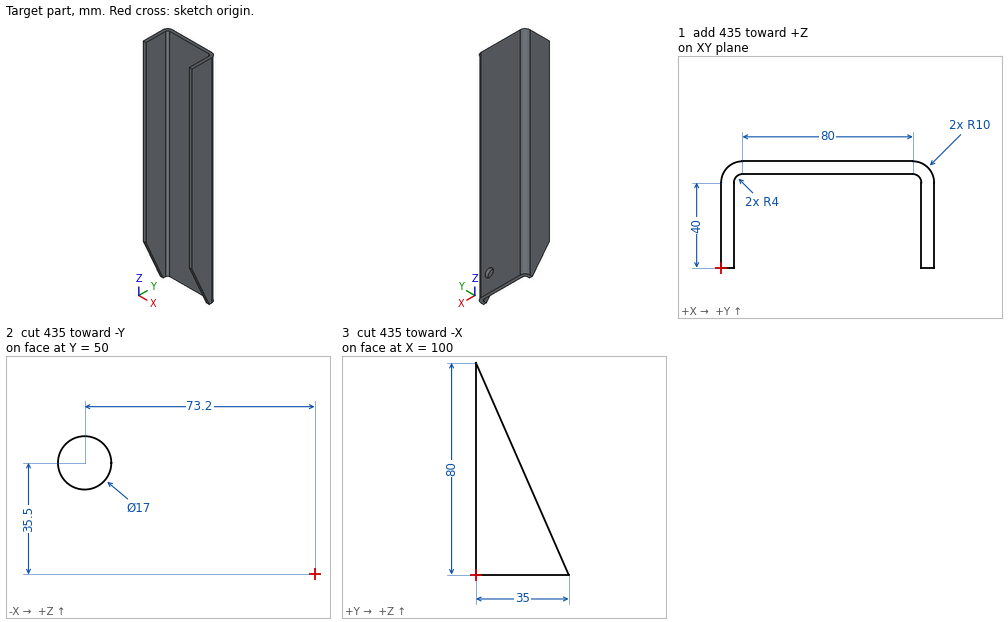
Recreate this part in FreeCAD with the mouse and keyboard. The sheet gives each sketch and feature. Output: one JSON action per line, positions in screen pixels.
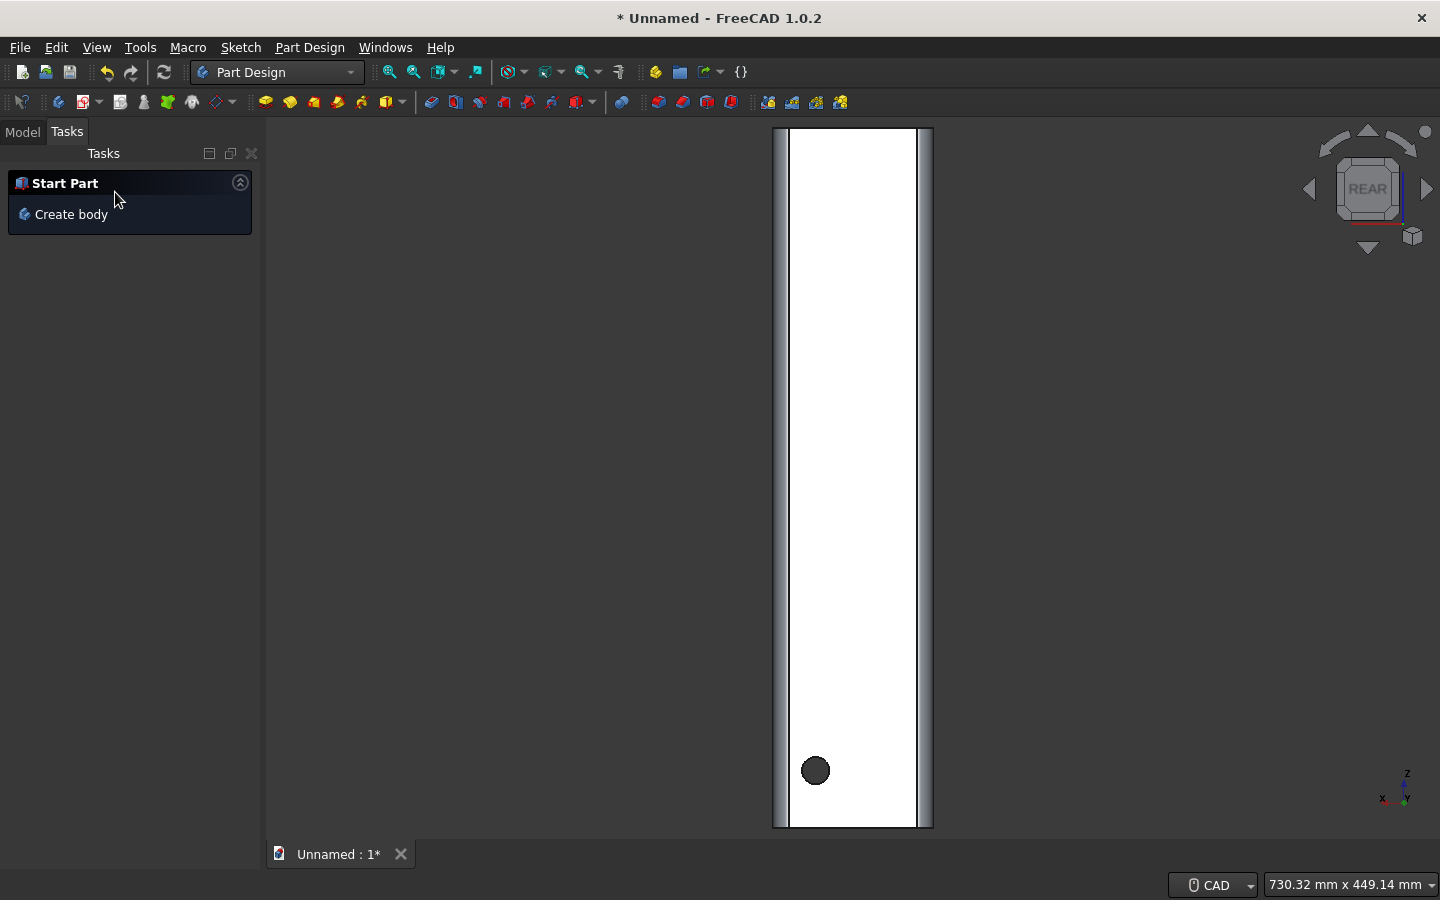
{"action": "key", "text": "0"}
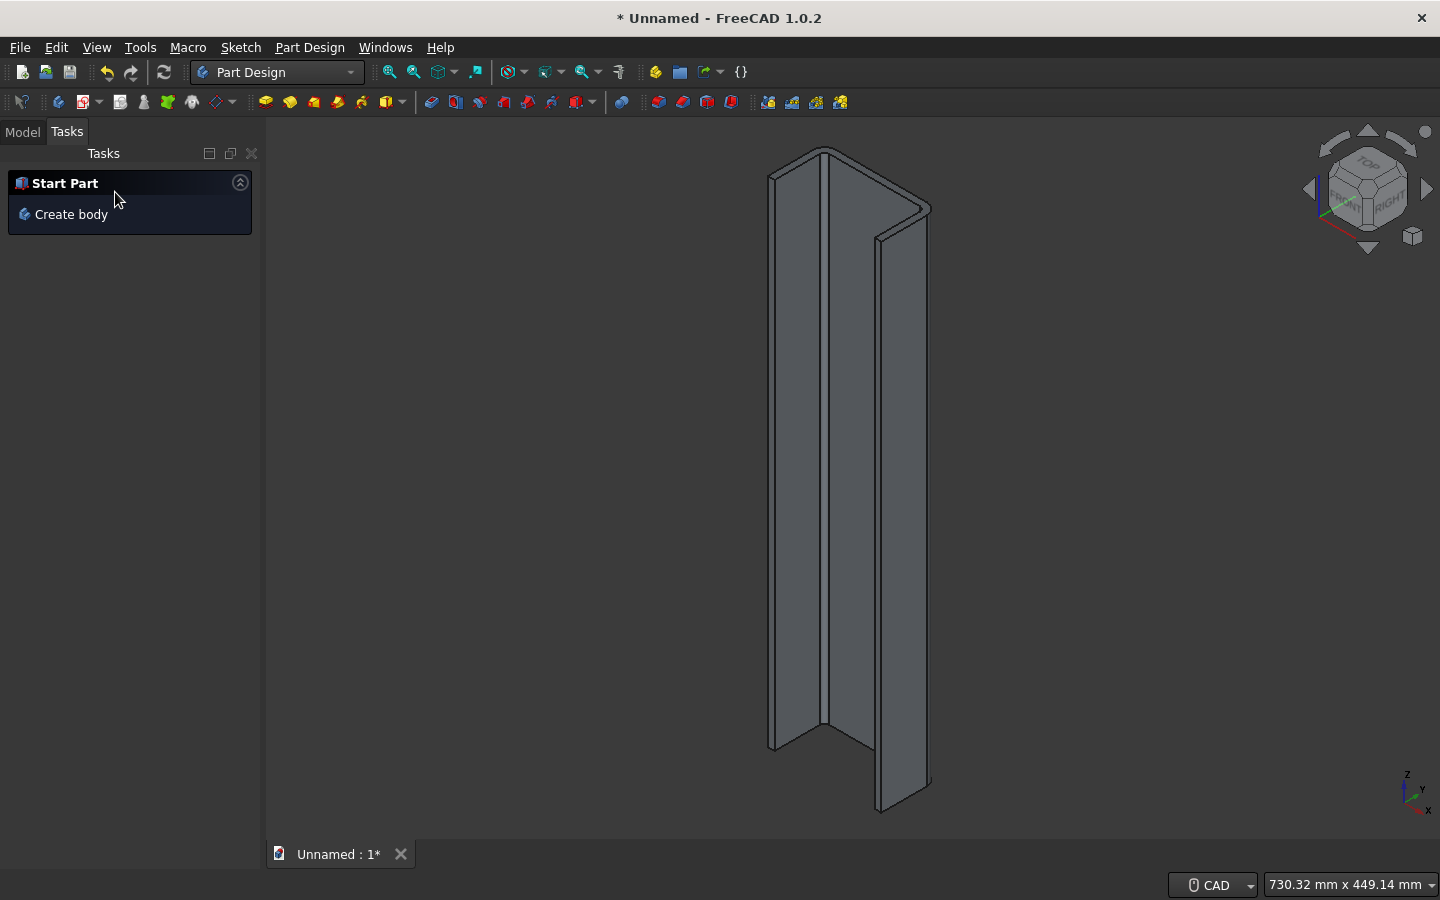
{"action": "left_click", "coordinate": [904, 268]}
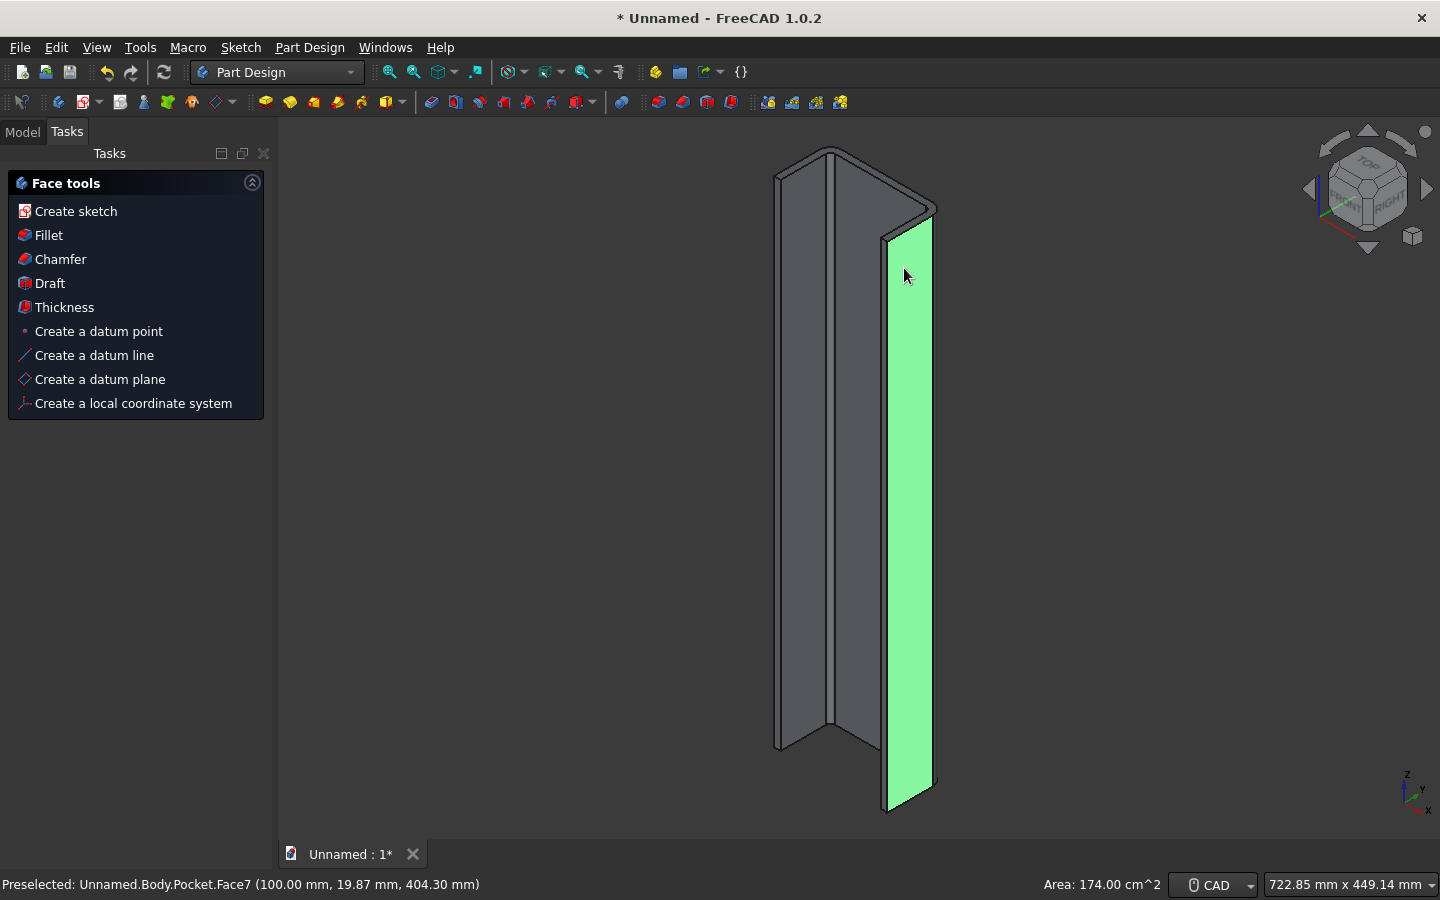
{"action": "left_click", "coordinate": [84, 102]}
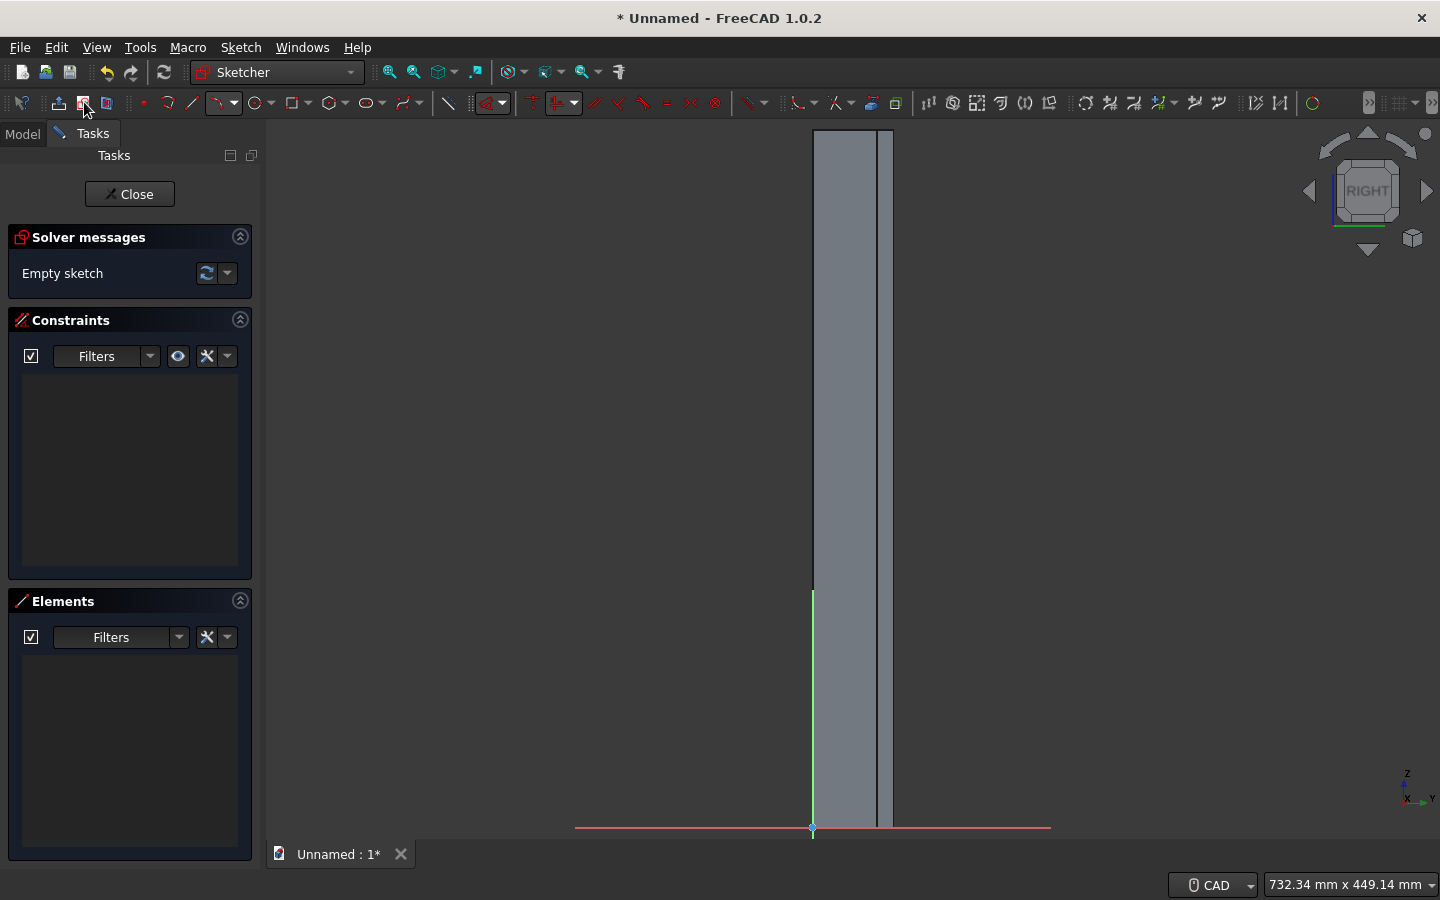
{"action": "scroll", "coordinate": [784, 479], "scroll_direction": "down", "scroll_amount": 5}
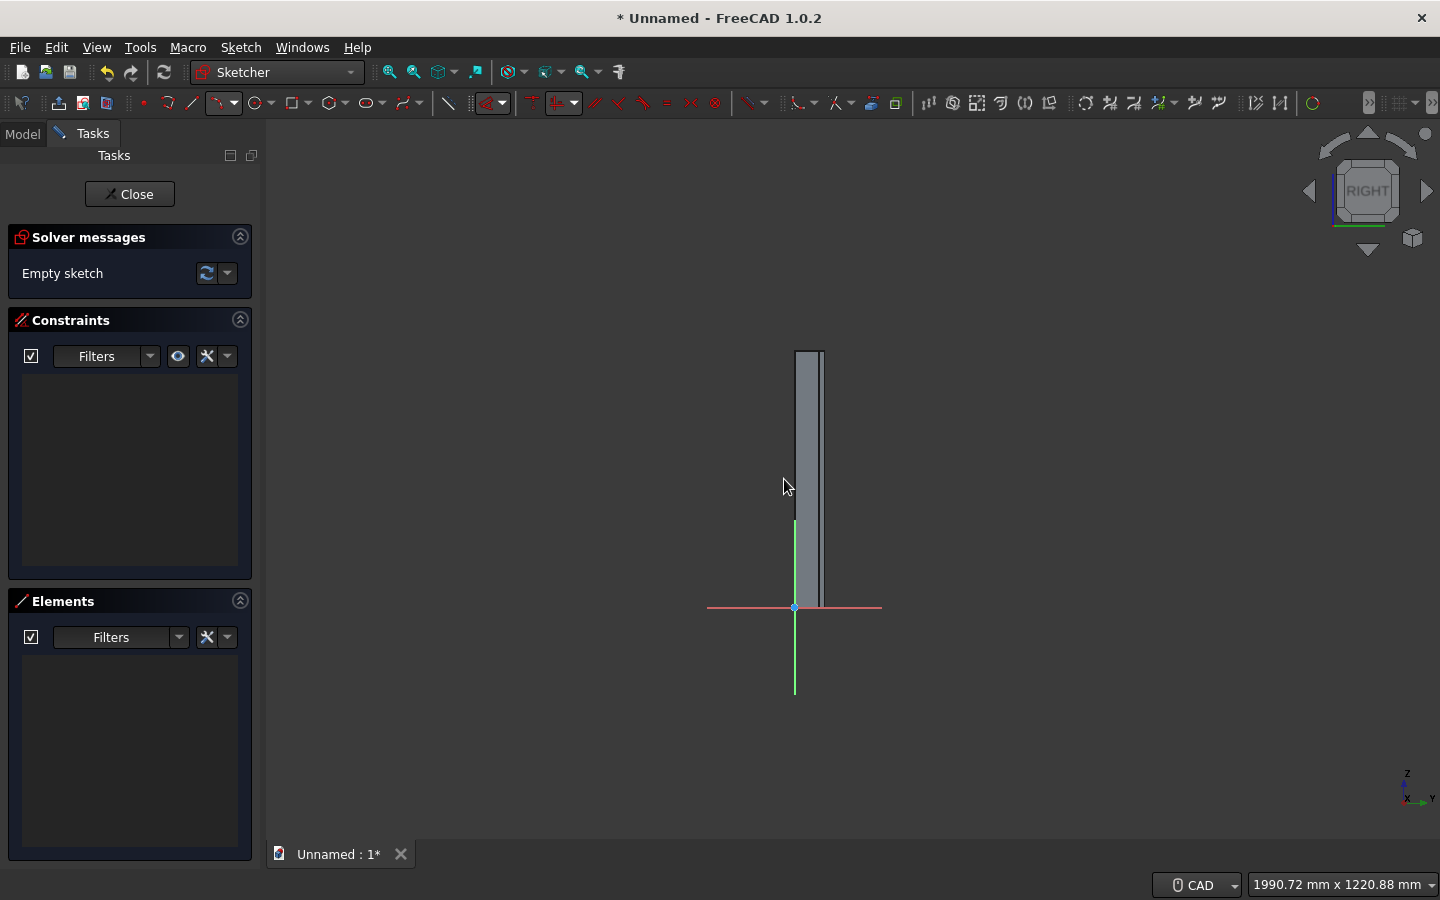
{"action": "scroll", "coordinate": [808, 597], "scroll_direction": "up", "scroll_amount": 11}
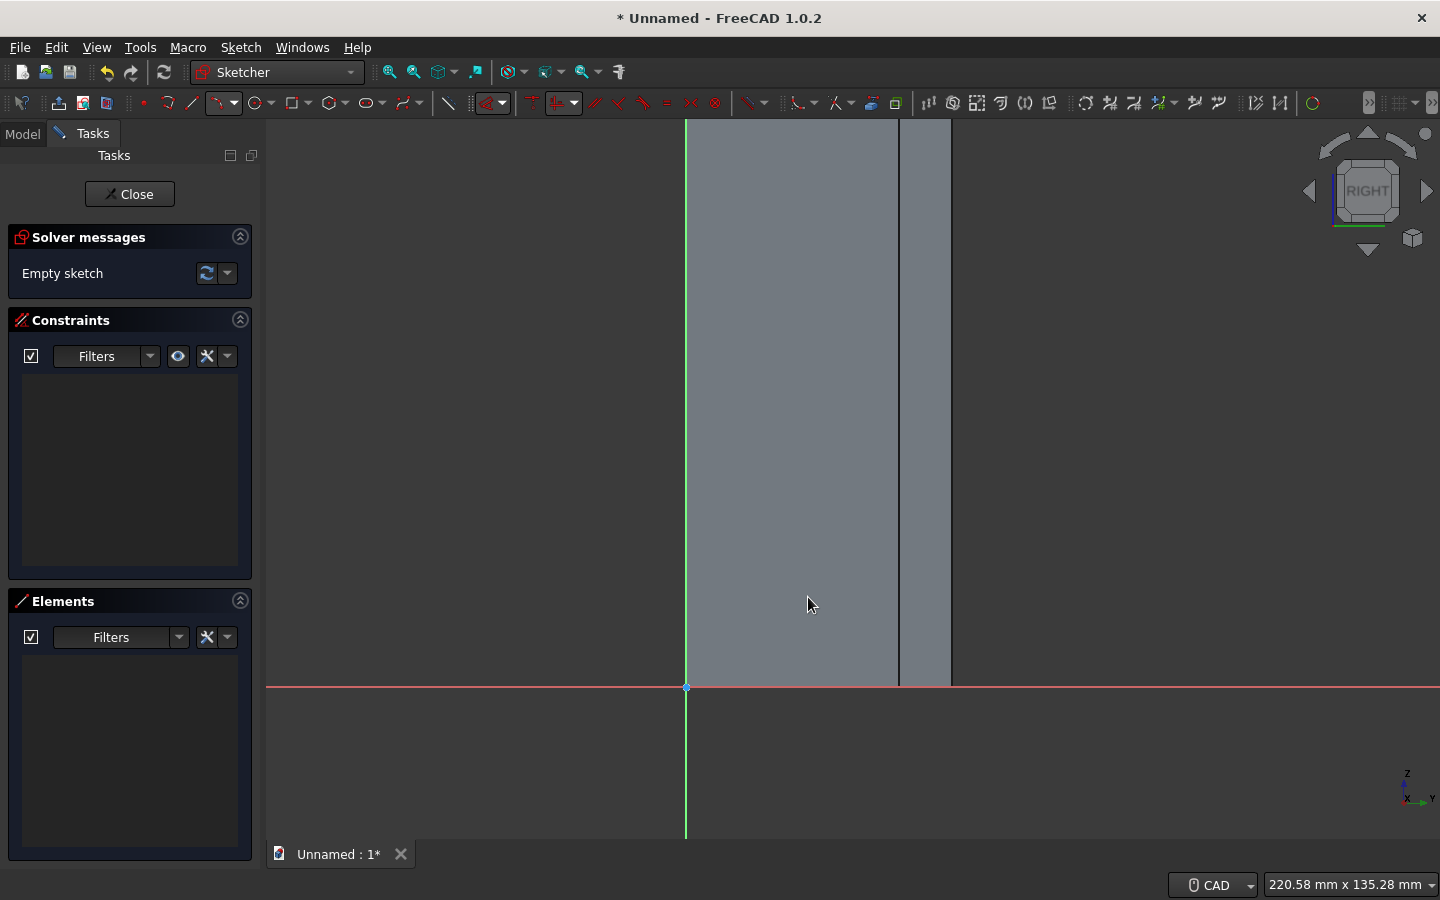
{"action": "left_click", "coordinate": [168, 104]}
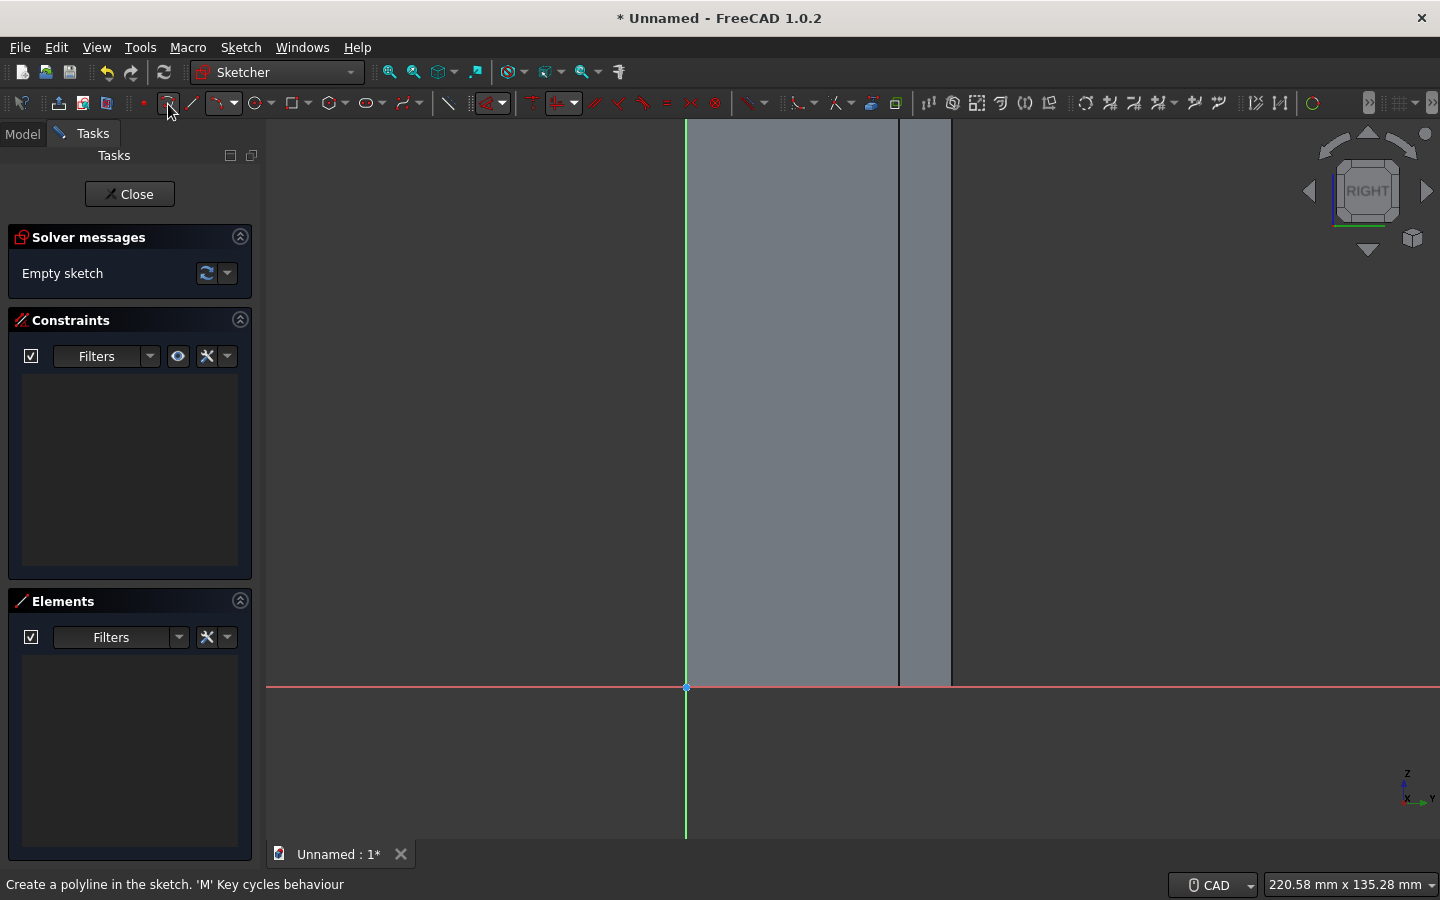
{"action": "left_click", "coordinate": [686, 687]}
{"action": "left_click", "coordinate": [873, 678]}
{"action": "left_click", "coordinate": [695, 261]}
{"action": "left_click", "coordinate": [686, 687]}
{"action": "key", "text": "Escape"}
{"action": "key", "text": "Escape"}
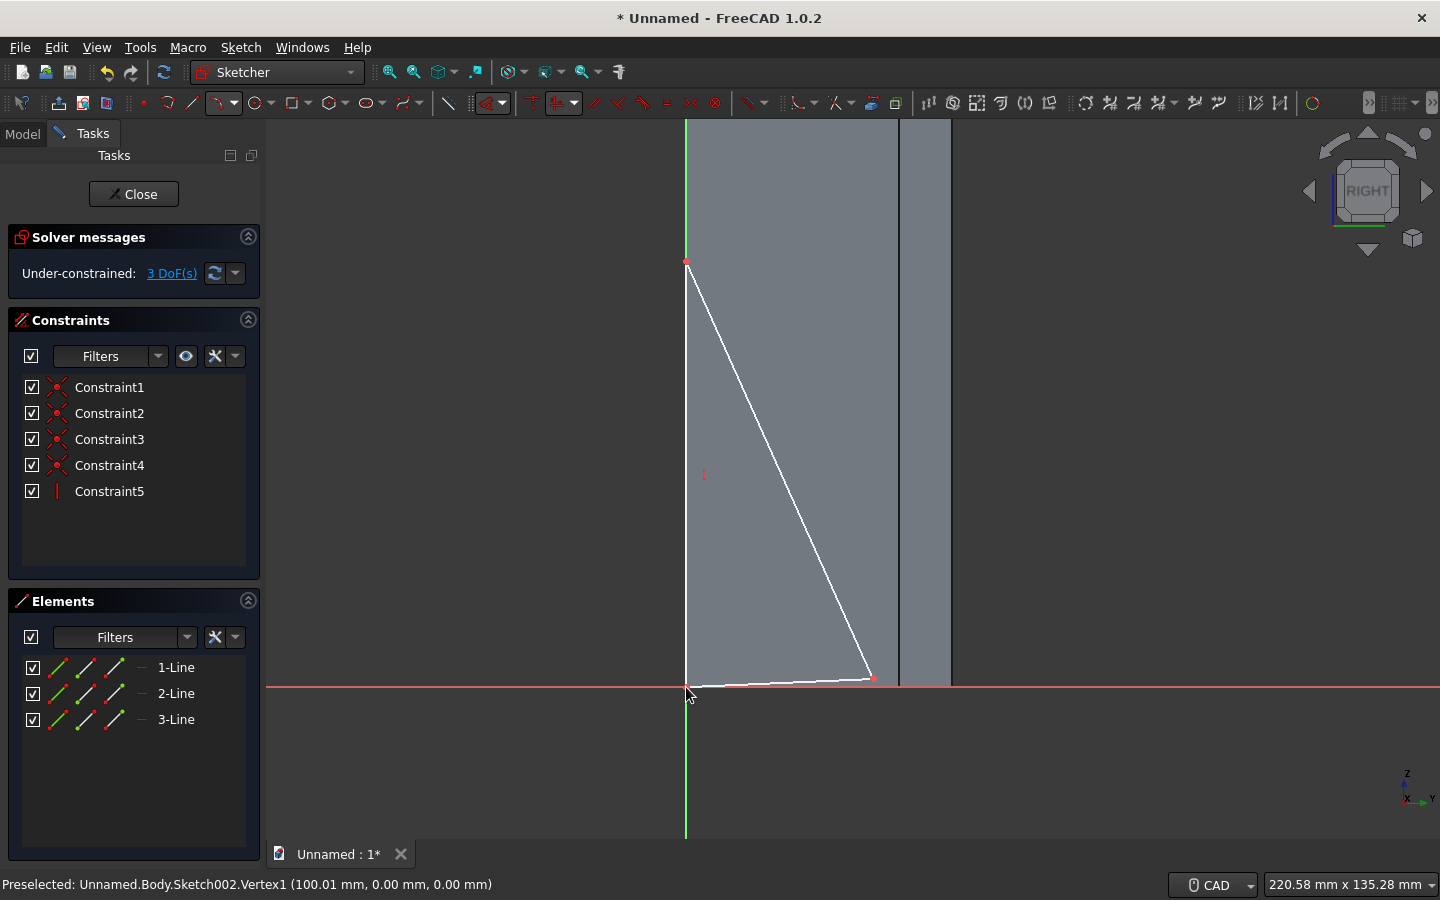
{"action": "left_click", "coordinate": [742, 685]}